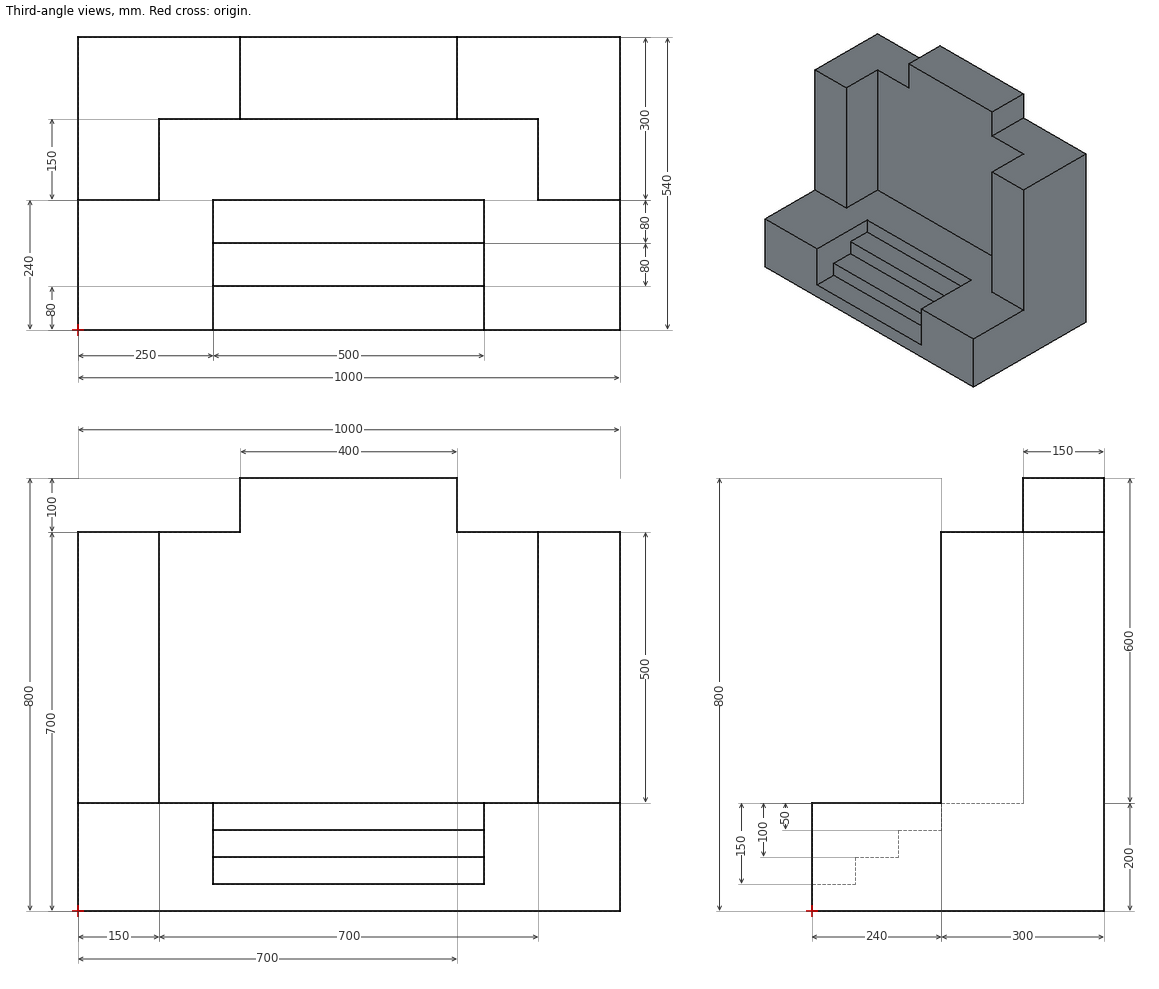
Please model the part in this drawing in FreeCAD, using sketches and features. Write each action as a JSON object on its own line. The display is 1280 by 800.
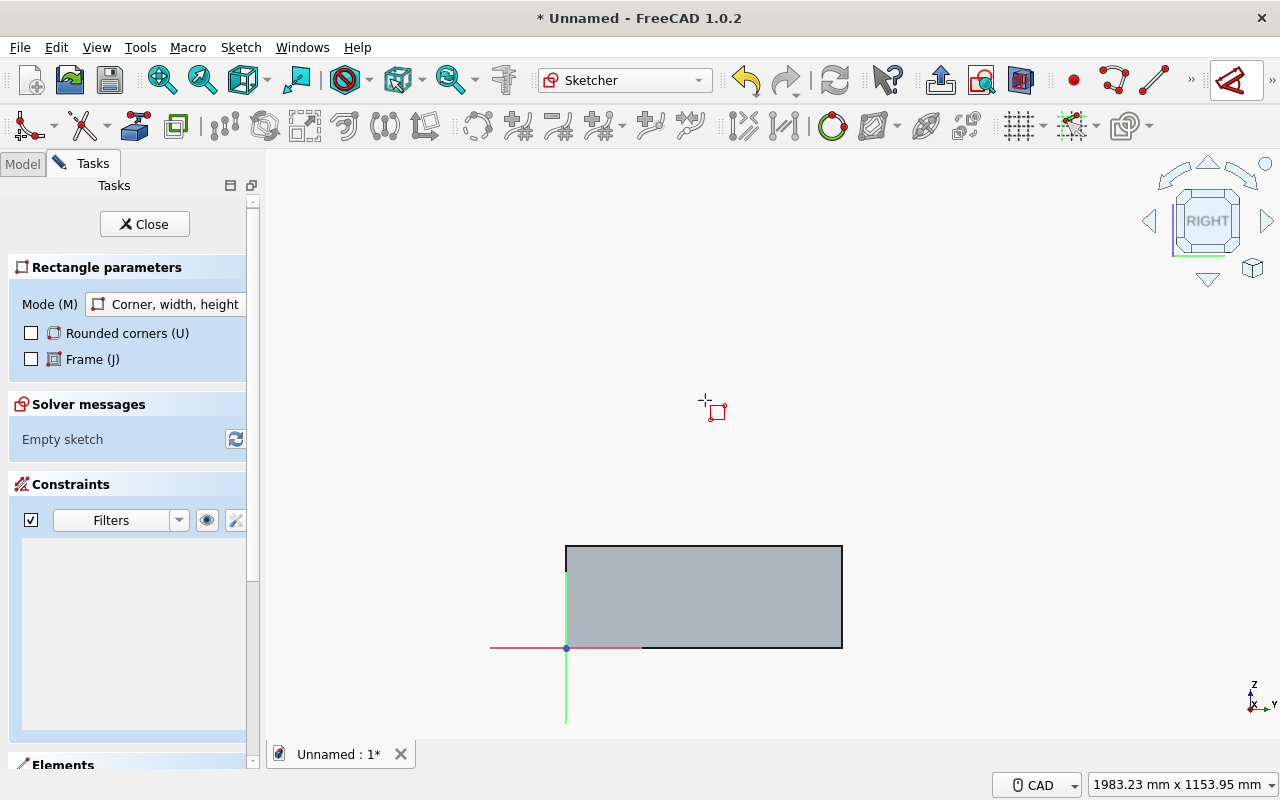
{"action": "left_click", "coordinate": [689, 239]}
{"action": "mouse_move", "coordinate": [842, 546]}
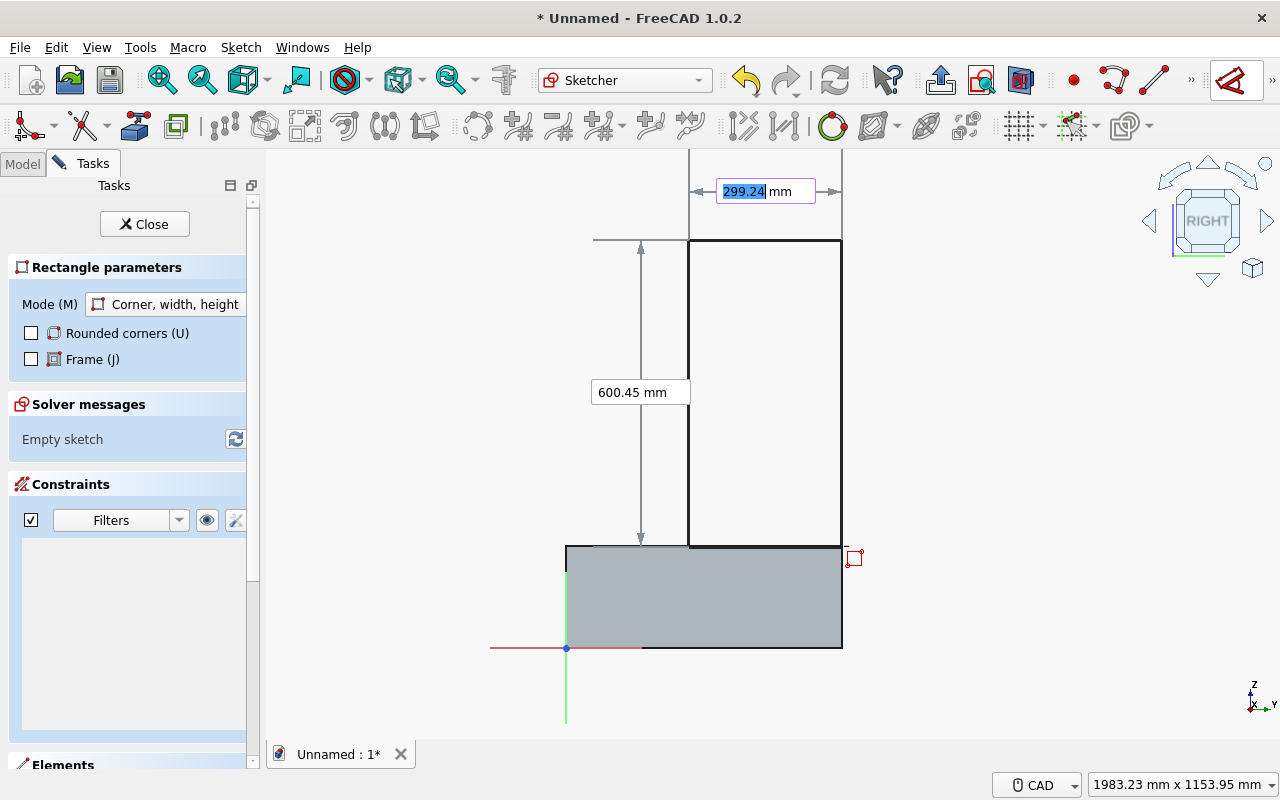
{"action": "type", "text": "300"}
{"action": "key", "text": "Tab"}
{"action": "type", "text": "600"}
{"action": "key", "text": "Return"}
{"action": "key", "text": "Escape"}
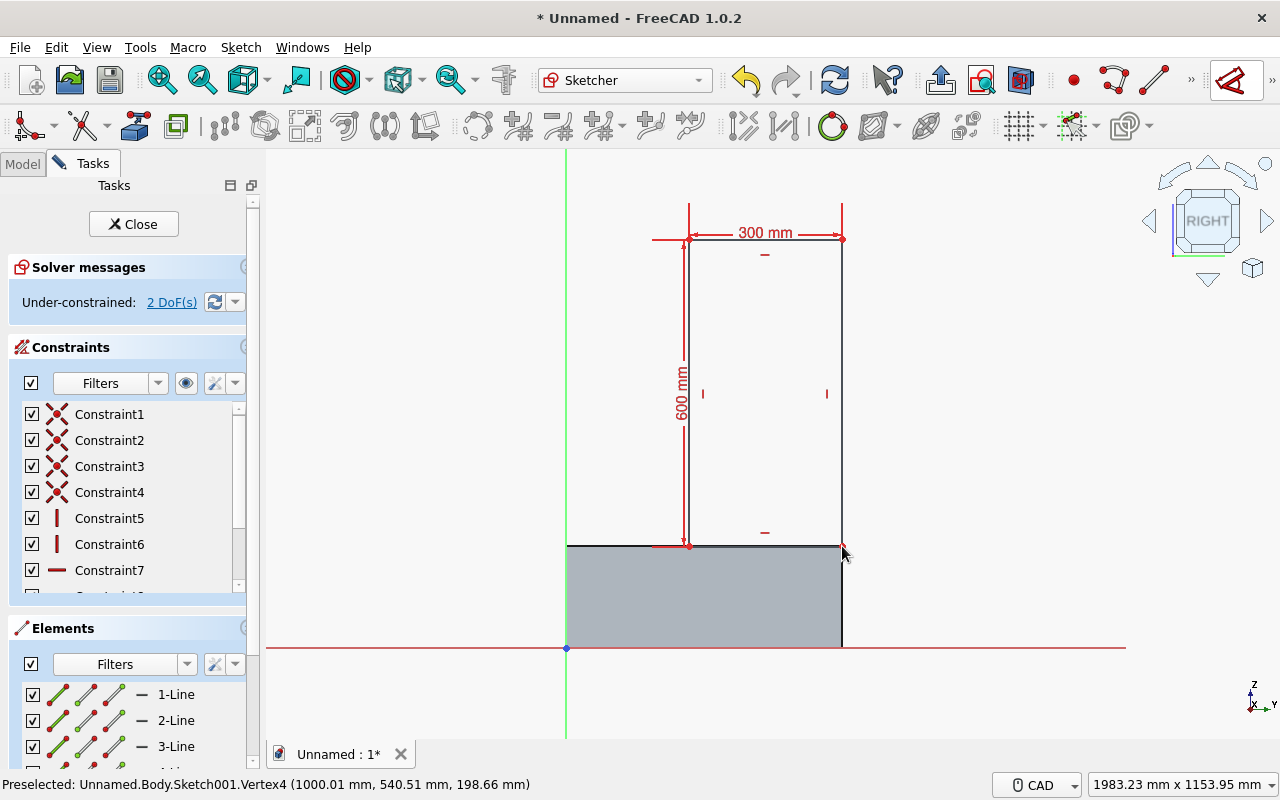
{"action": "left_click", "coordinate": [1230, 80]}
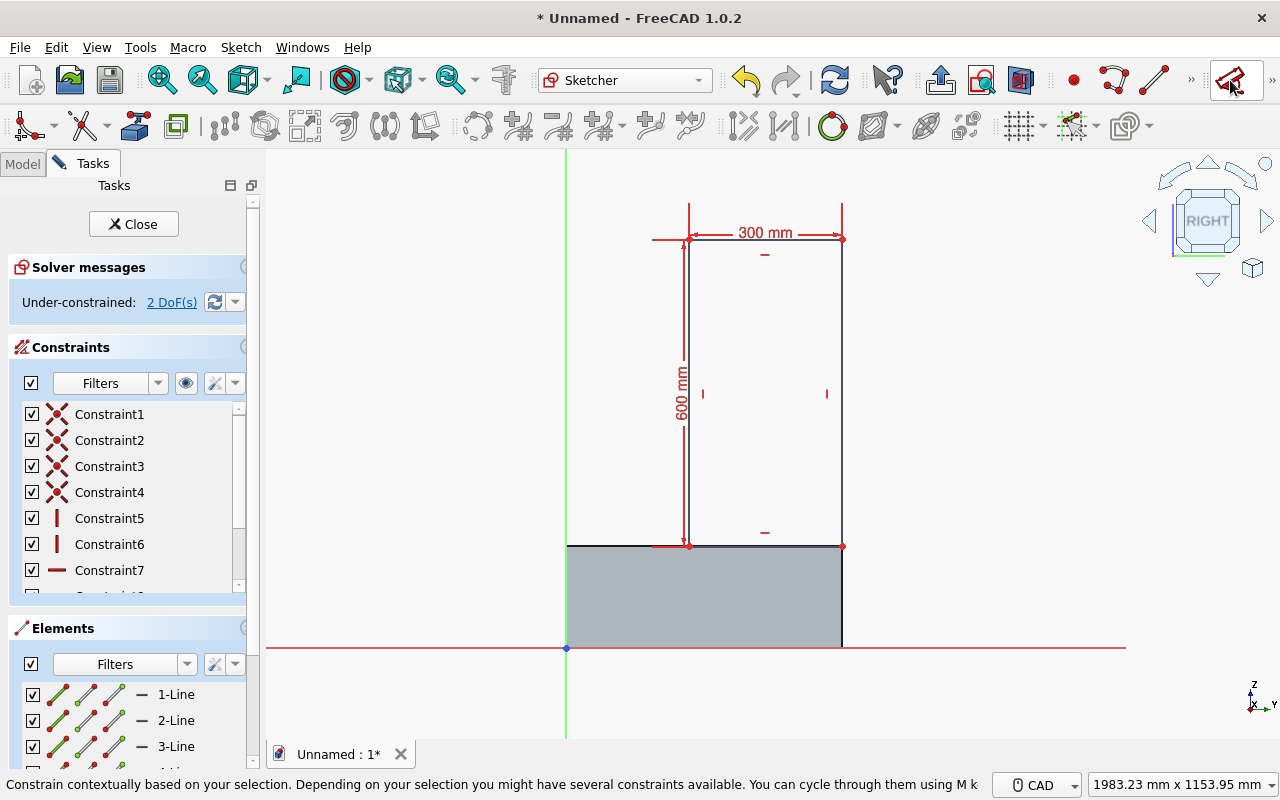
{"action": "left_click", "coordinate": [689, 240]}
{"action": "left_click", "coordinate": [628, 682]}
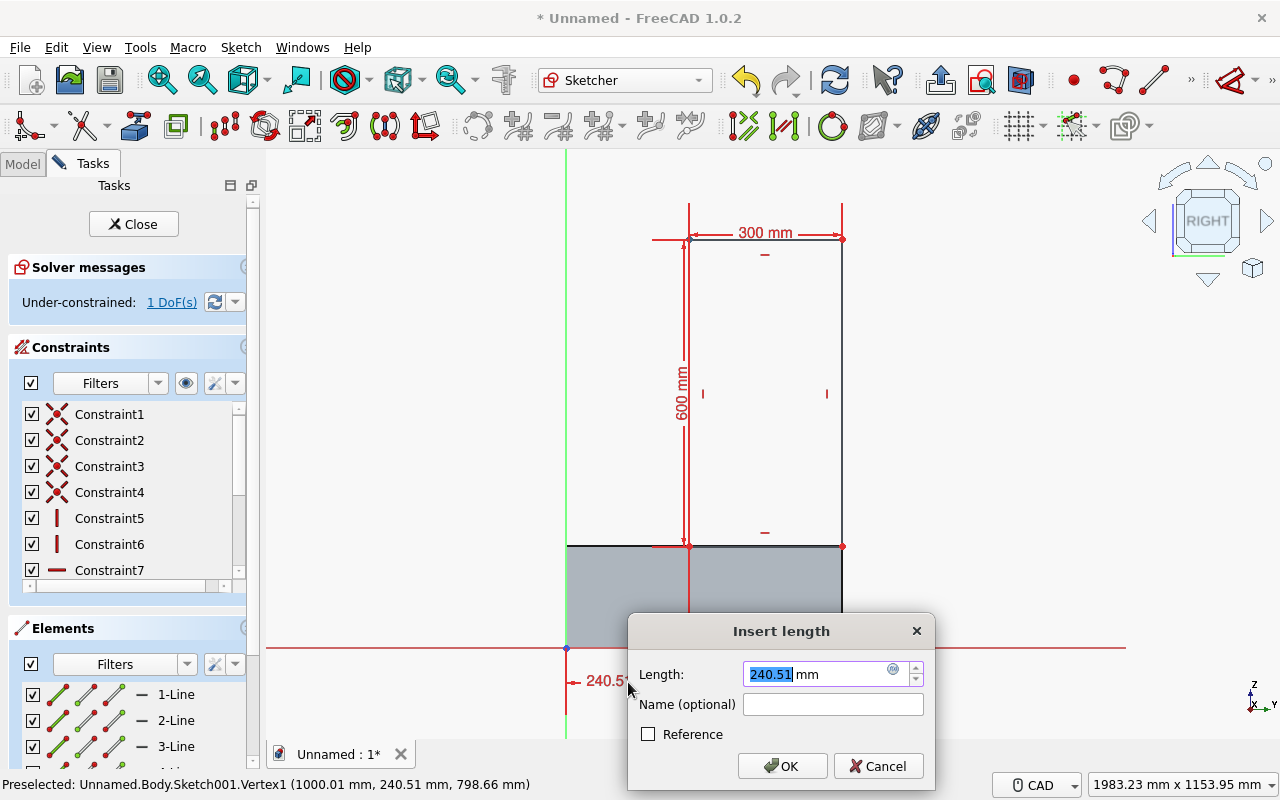
{"action": "type", "text": "240"}
{"action": "key", "text": "Return"}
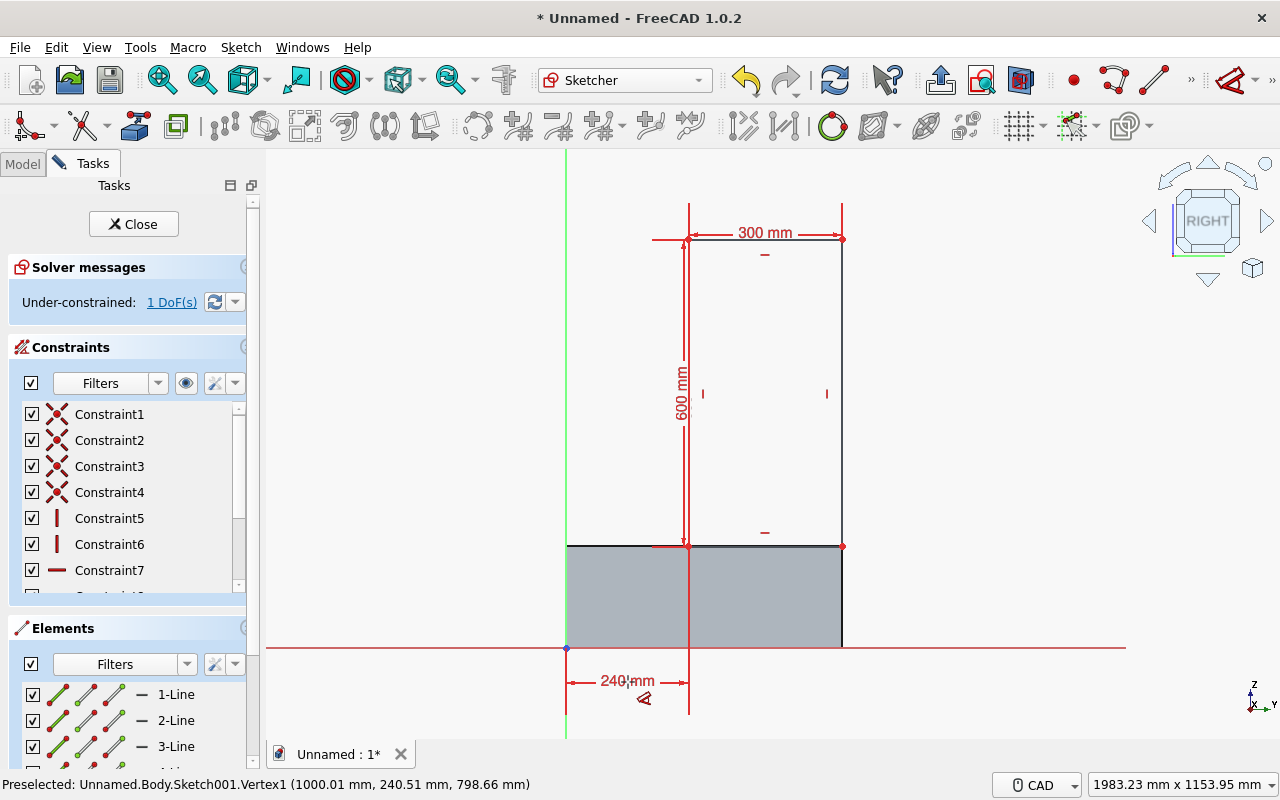
{"action": "left_click", "coordinate": [689, 240]}
{"action": "left_click", "coordinate": [532, 444]}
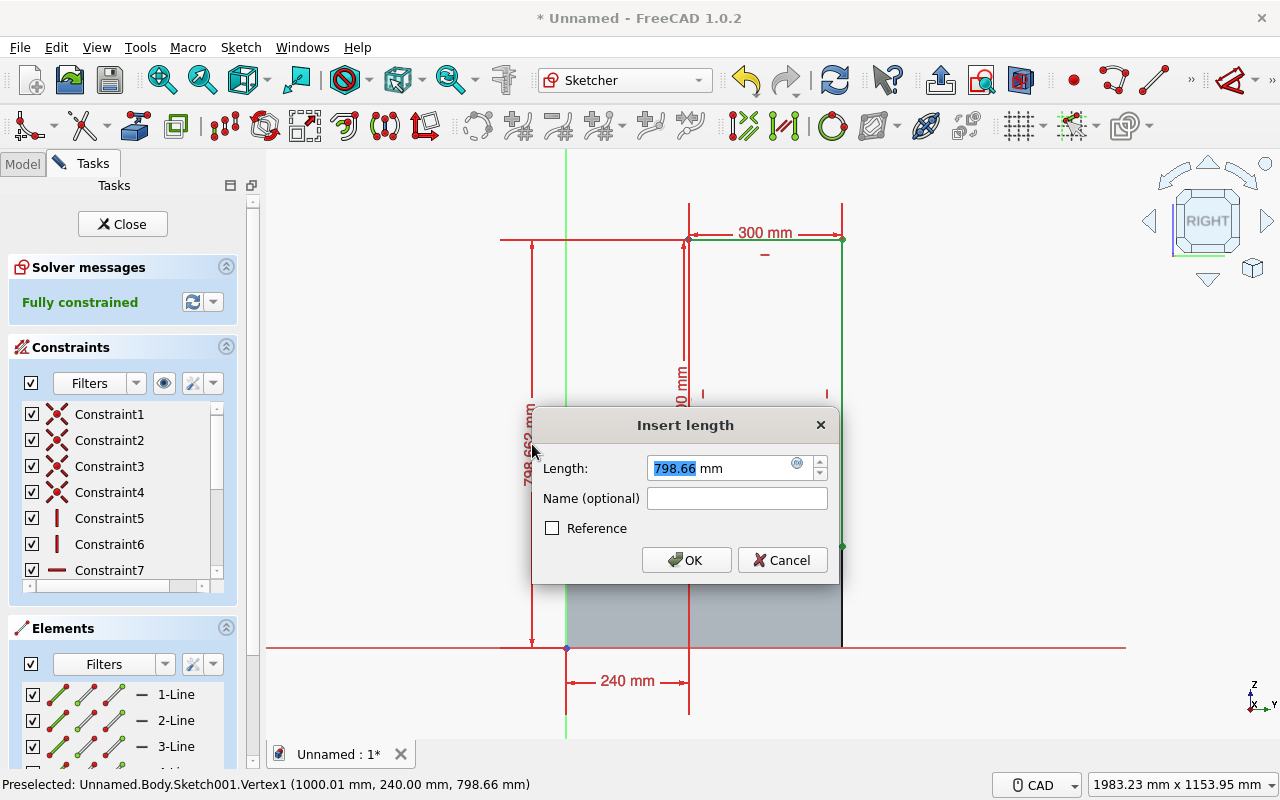
{"action": "type", "text": "800"}
{"action": "key", "text": "Return"}
{"action": "key", "text": "Escape"}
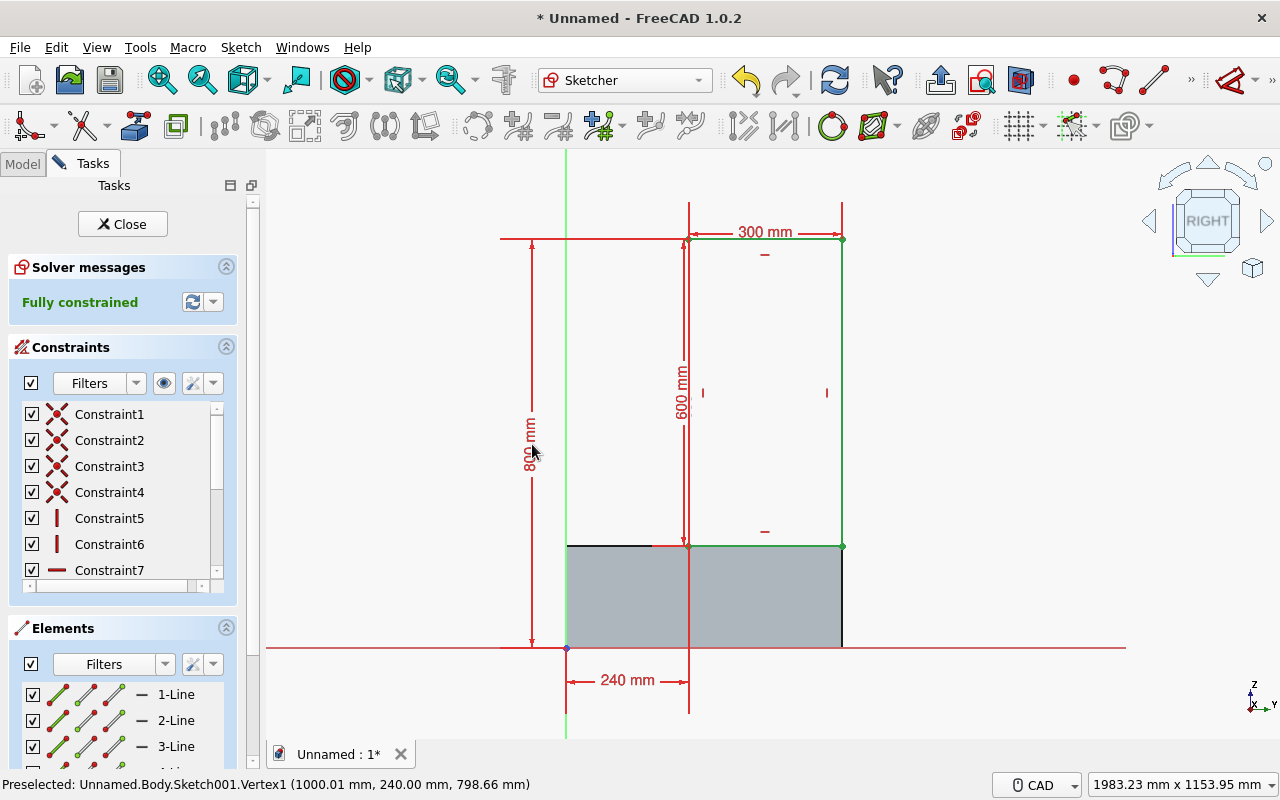
{"action": "left_click", "coordinate": [123, 224]}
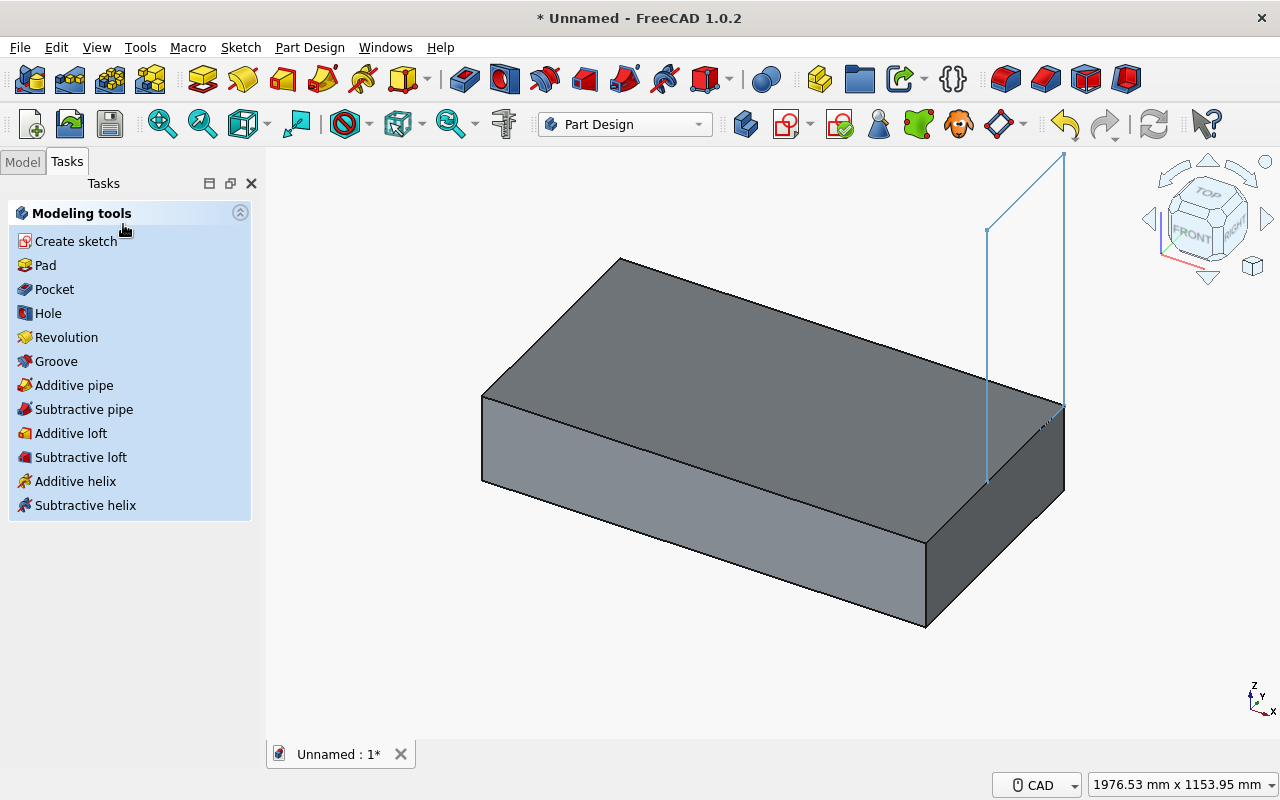
{"action": "left_click", "coordinate": [204, 80]}